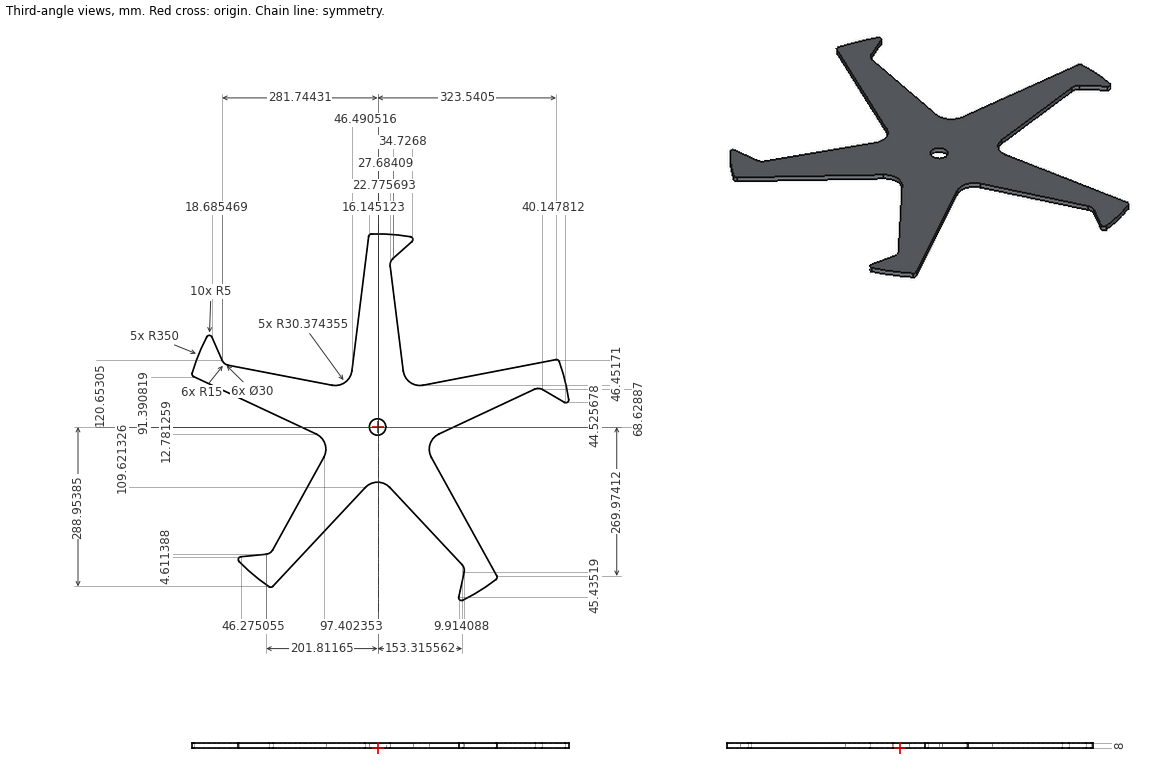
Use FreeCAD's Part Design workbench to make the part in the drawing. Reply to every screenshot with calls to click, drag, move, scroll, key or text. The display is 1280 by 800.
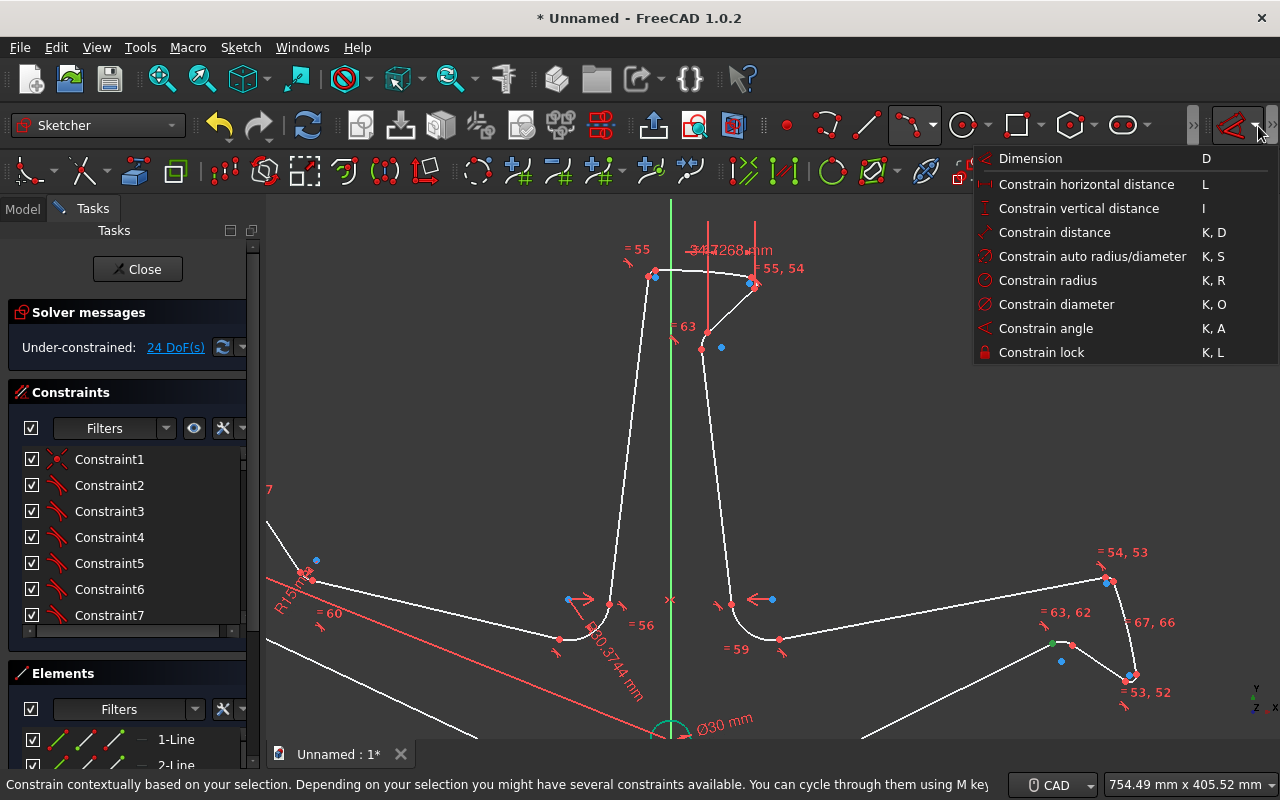
click(1126, 208)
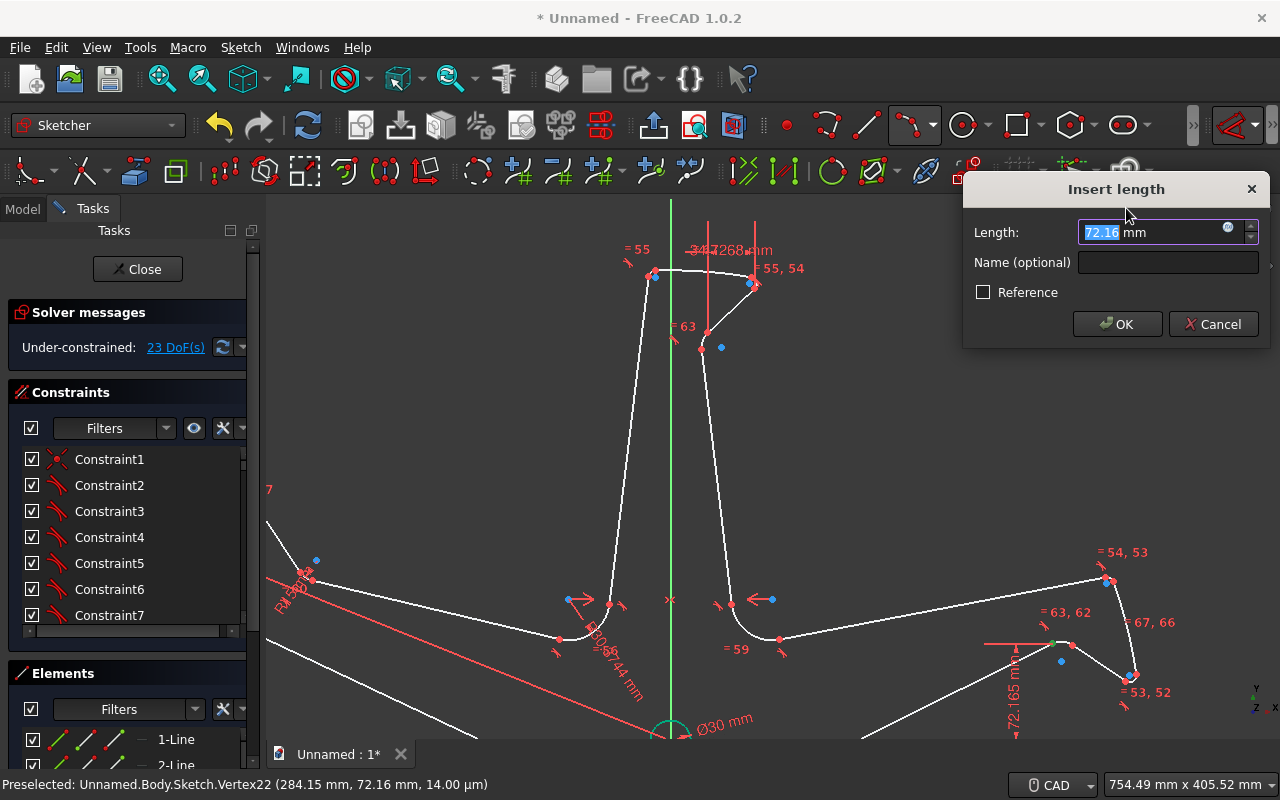
text(68.62887)
key(Return)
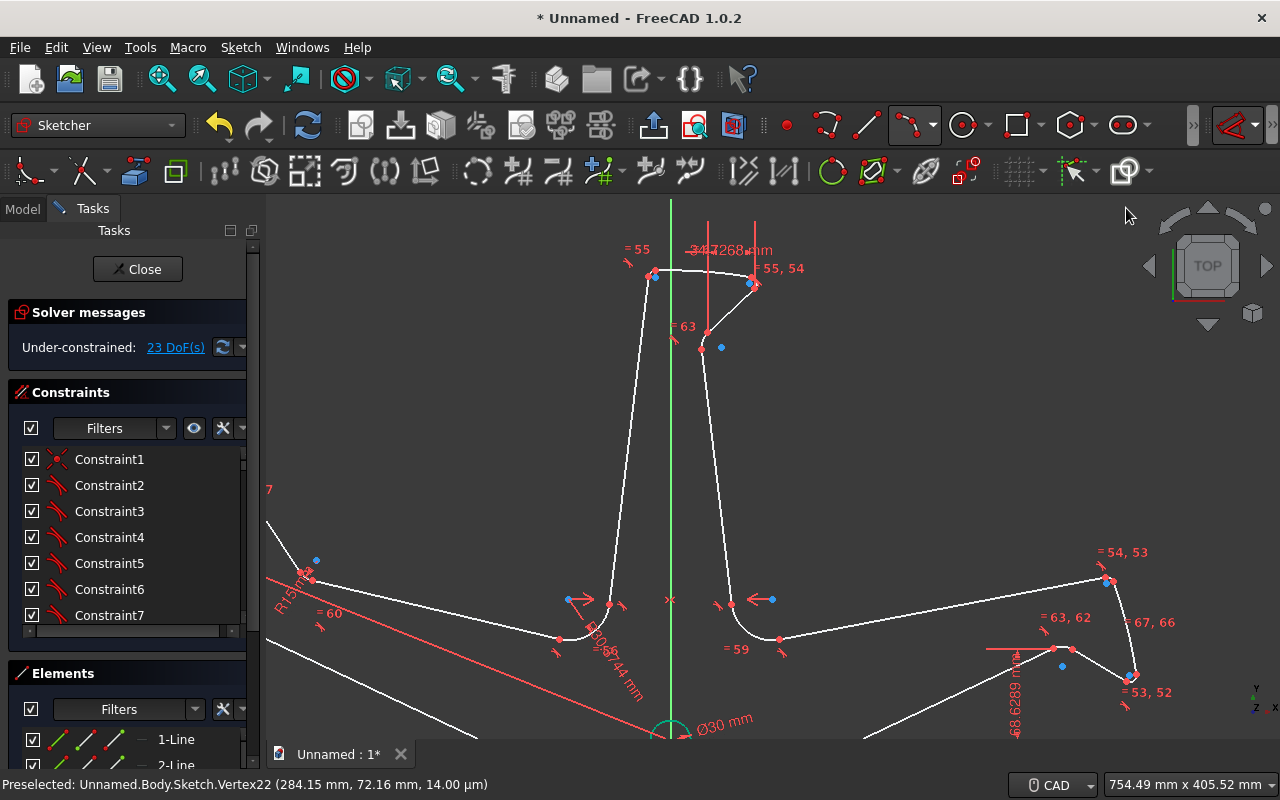
scroll(1106, 577, up, 3)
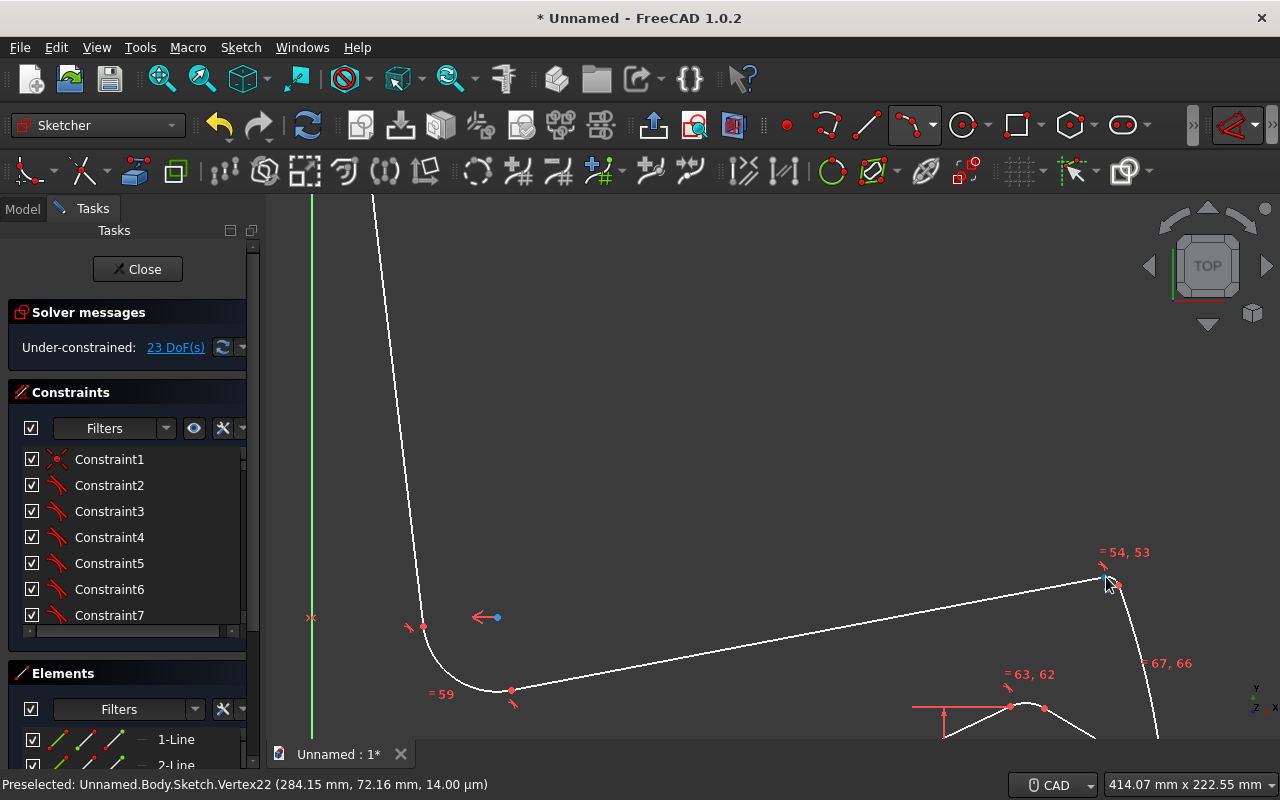
click(1105, 577)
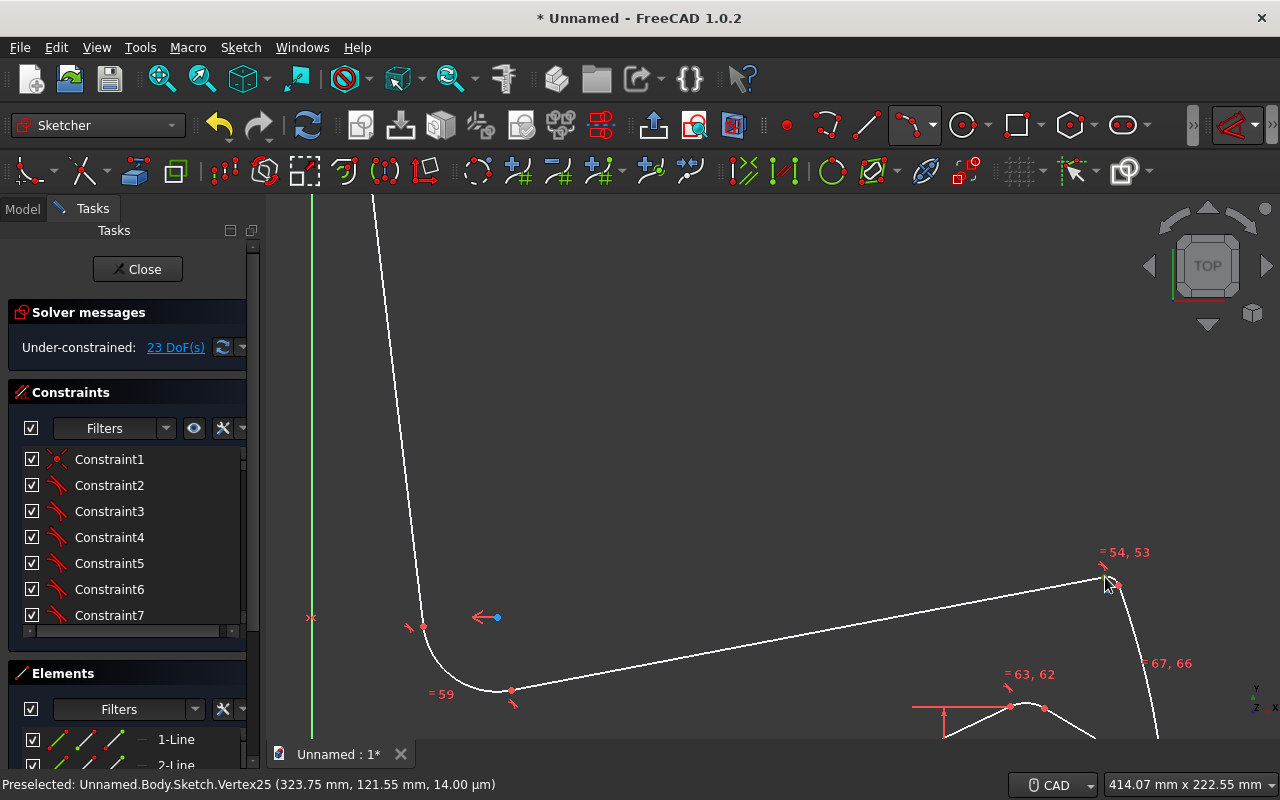
key(l)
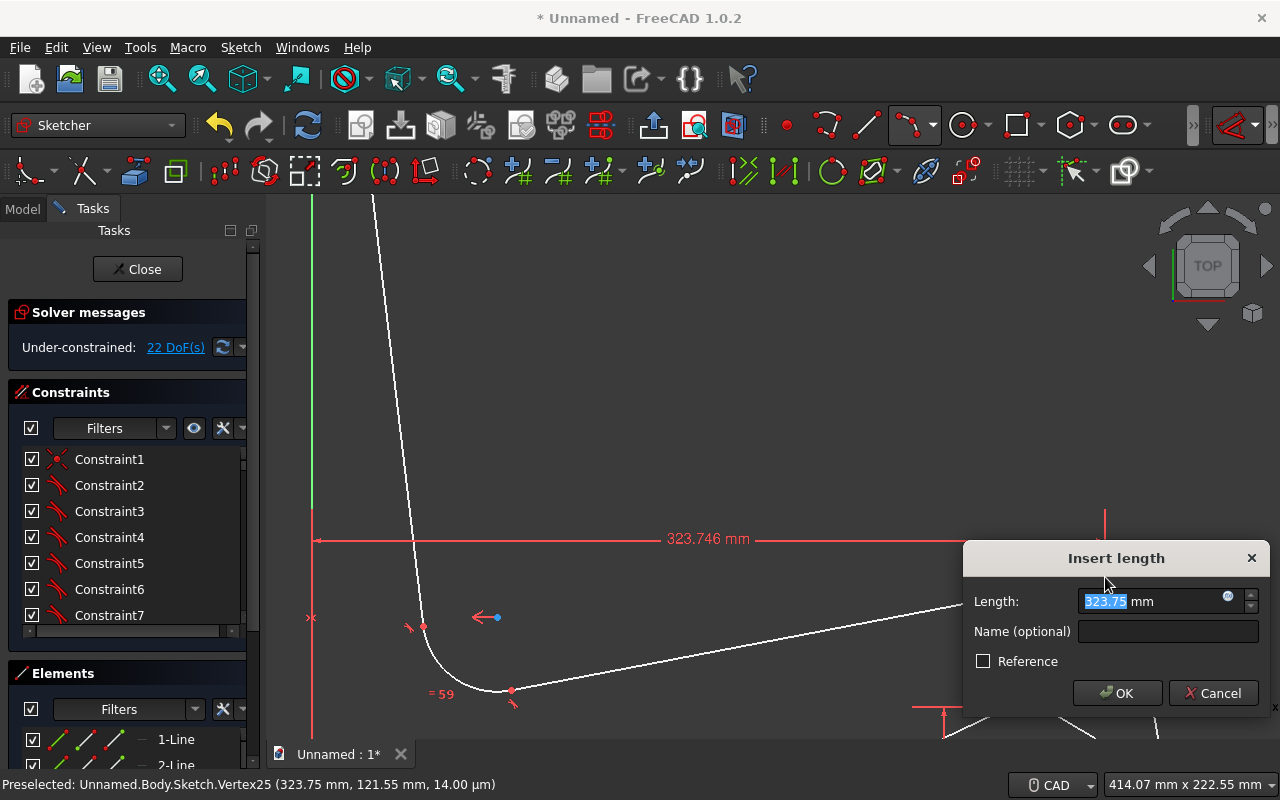
text(323.5405)
key(Return)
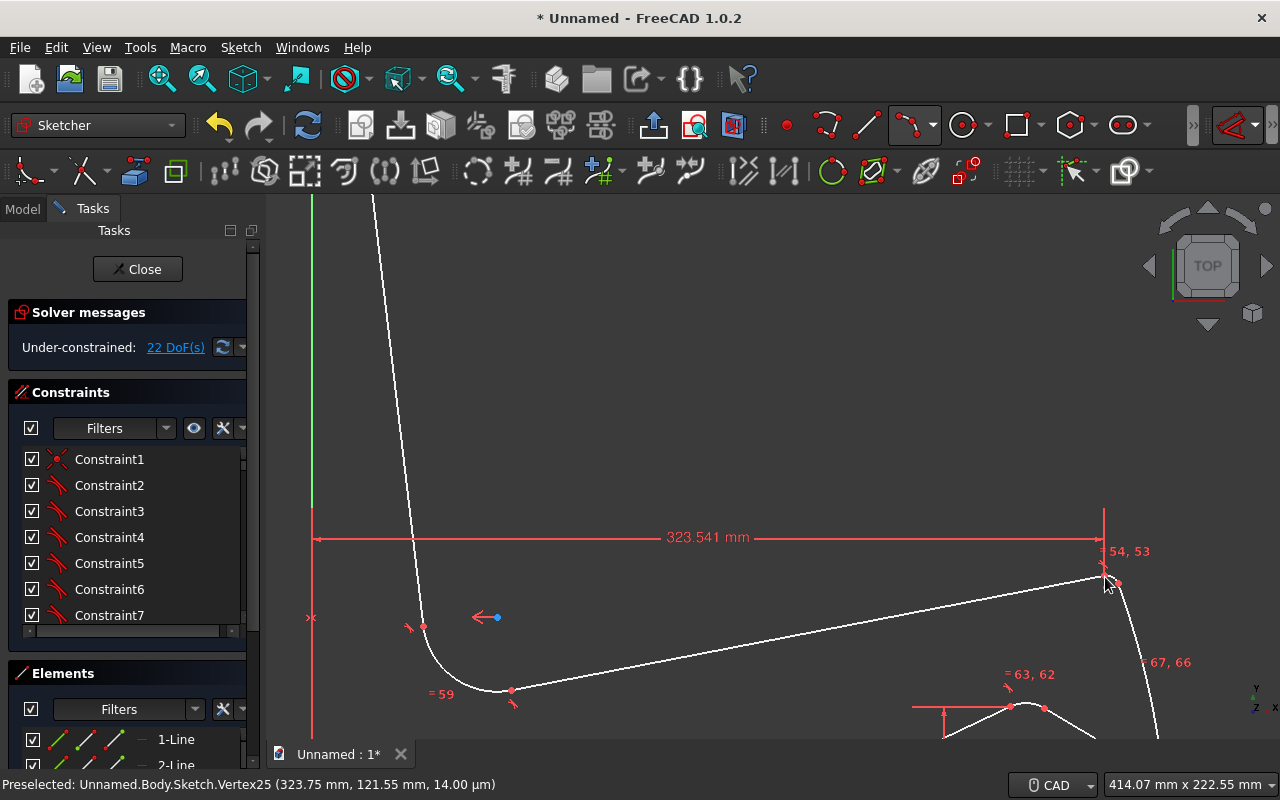
scroll(801, 374, down, 8)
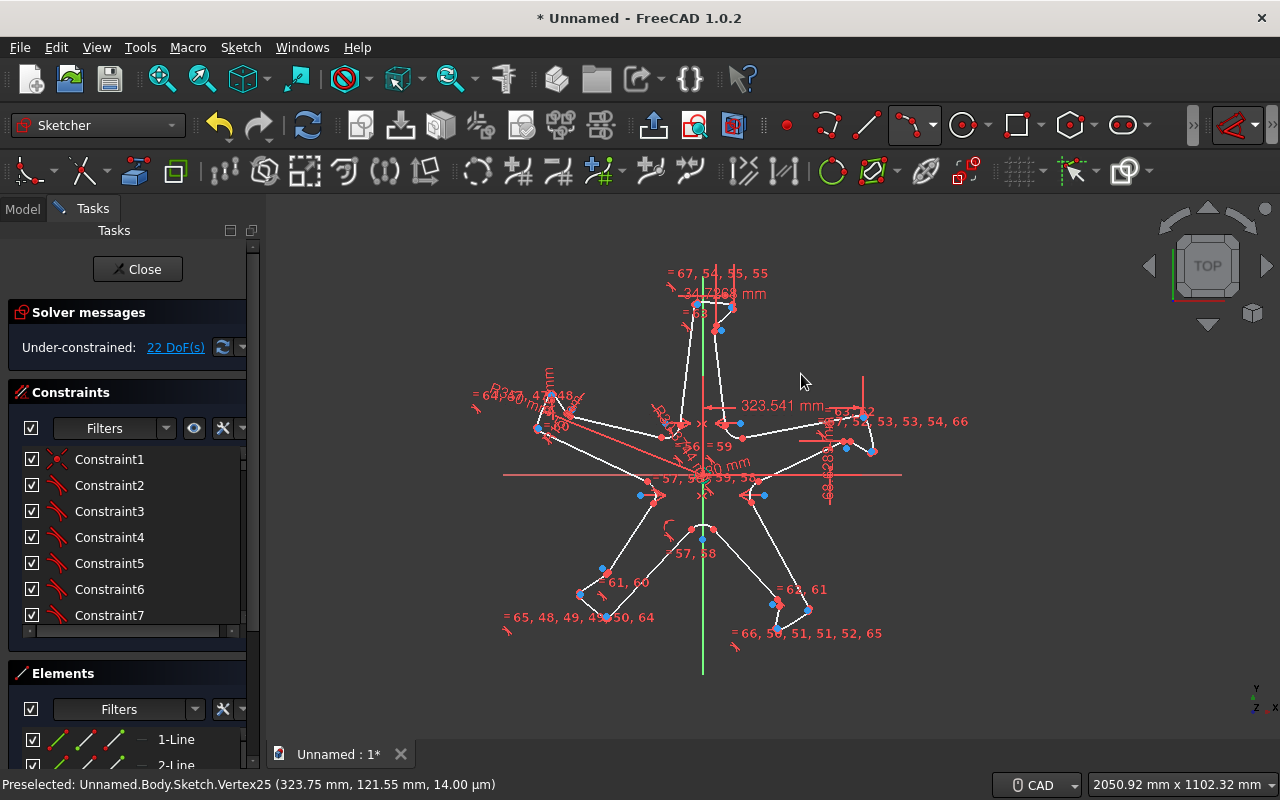
scroll(716, 325, up, 6)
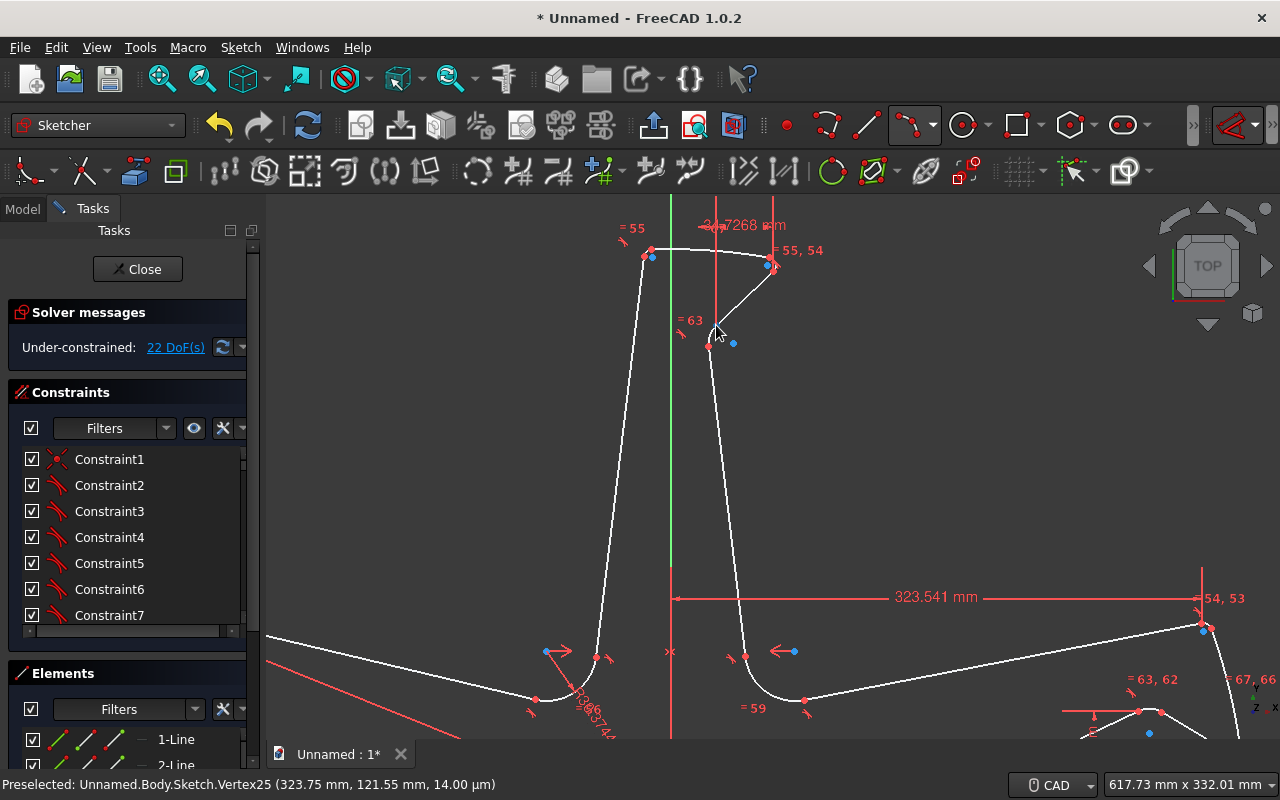
click(716, 326)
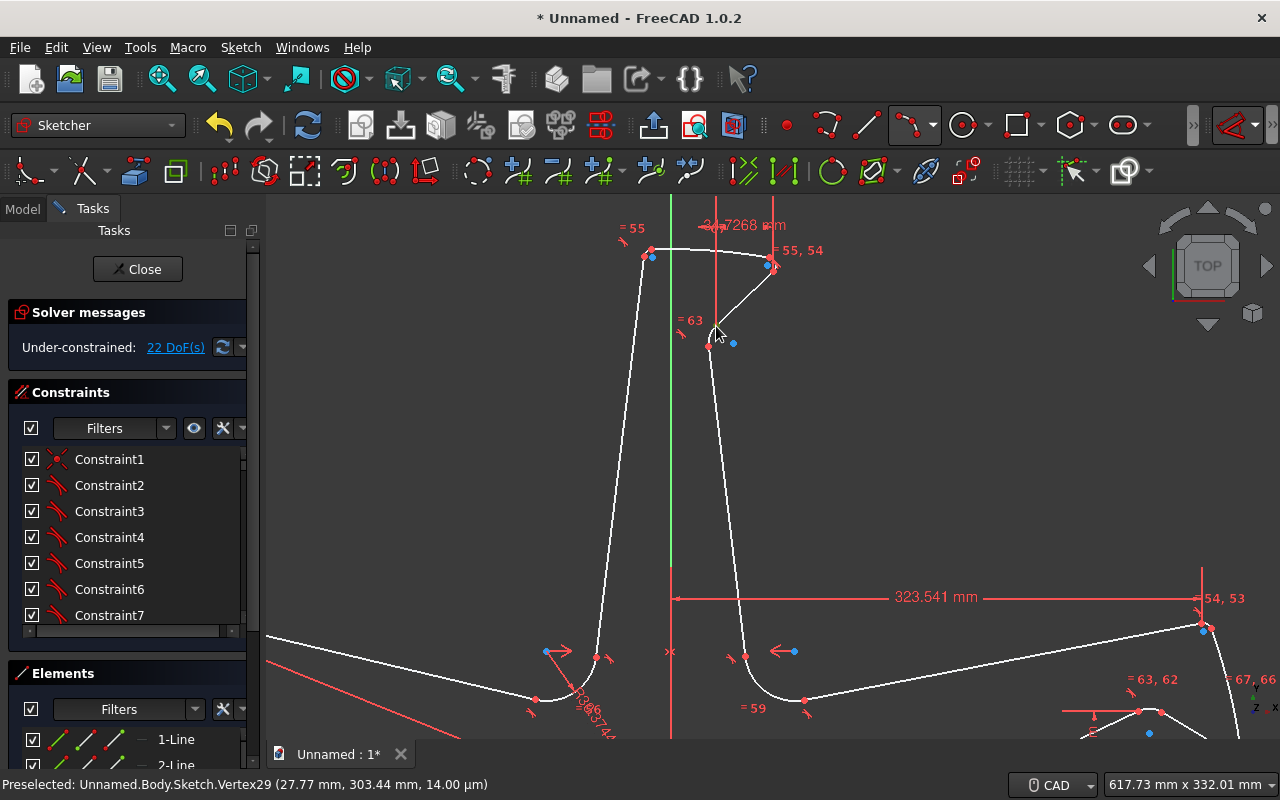
click(1258, 126)